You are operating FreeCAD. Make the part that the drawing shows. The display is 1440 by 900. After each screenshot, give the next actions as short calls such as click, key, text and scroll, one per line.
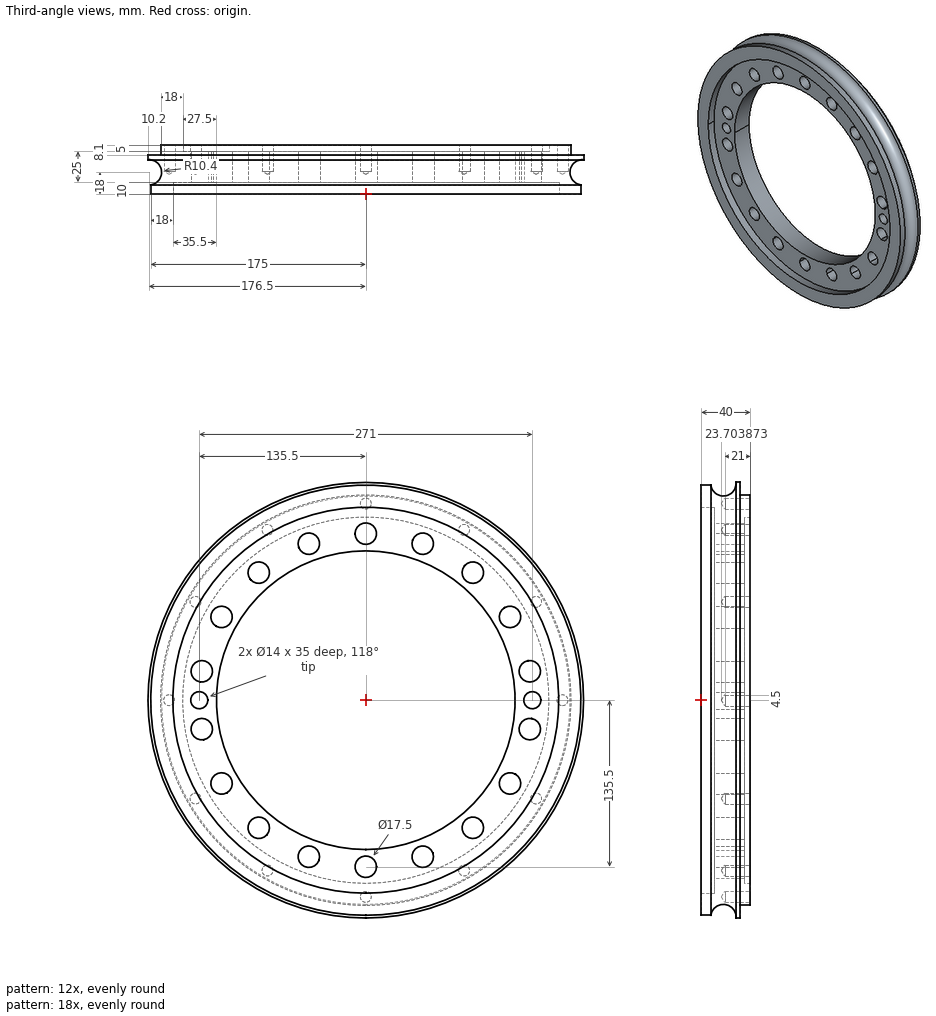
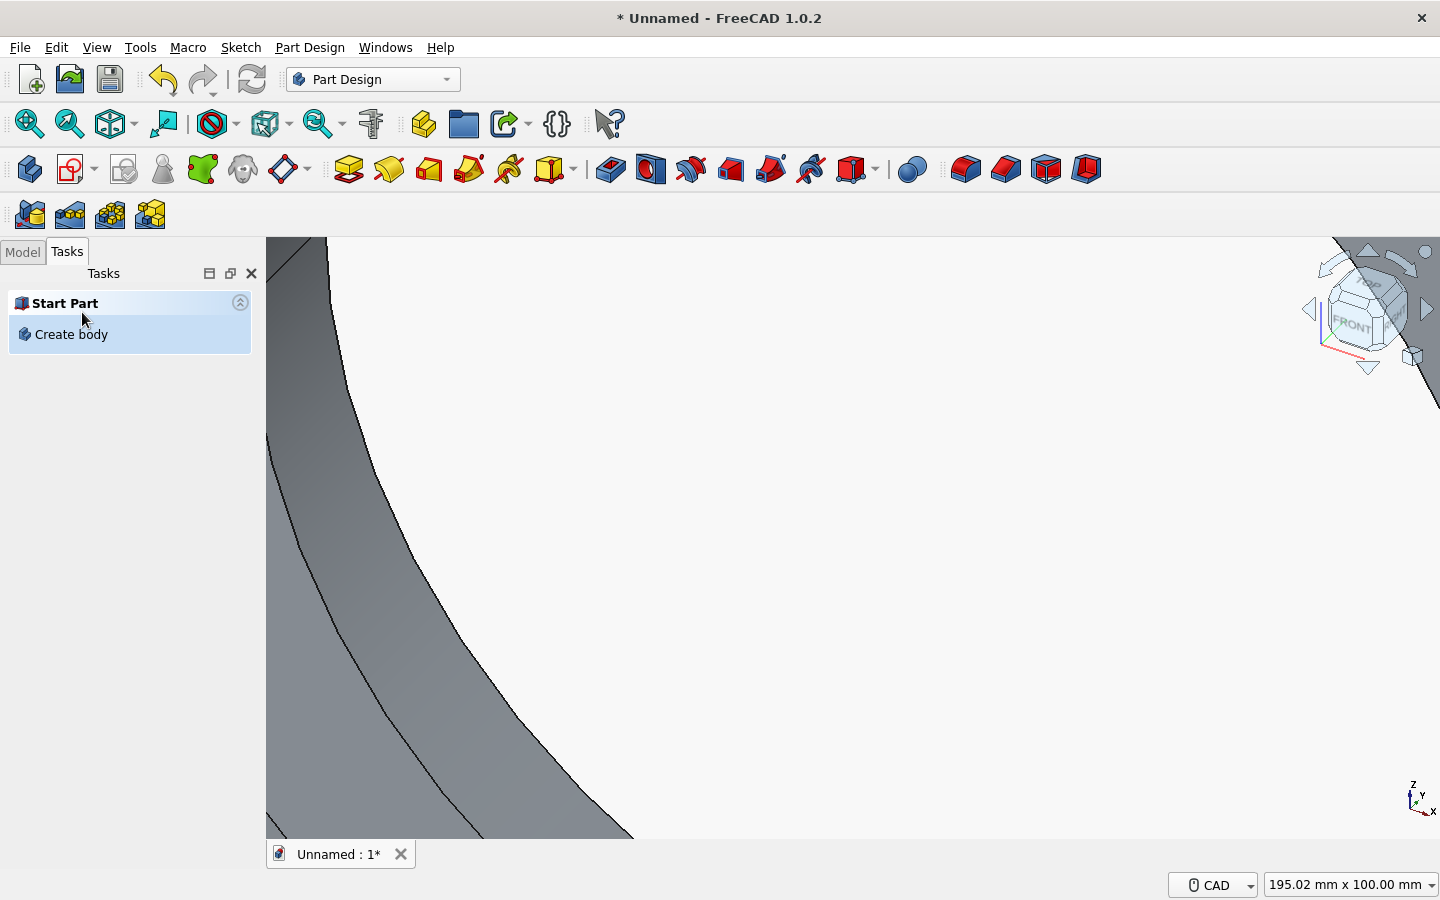
click(30, 124)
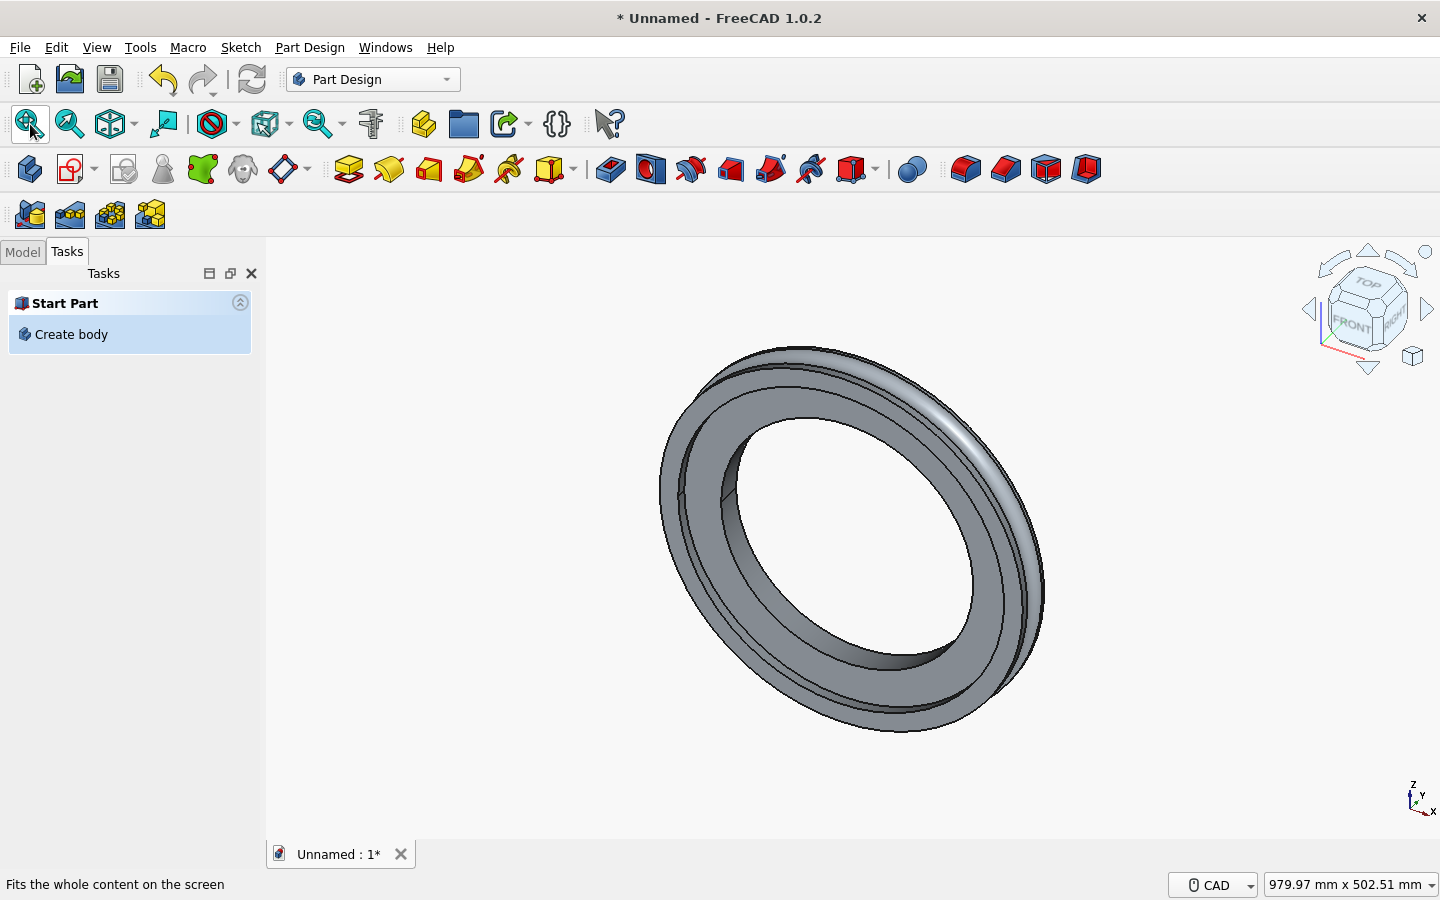
click(23, 251)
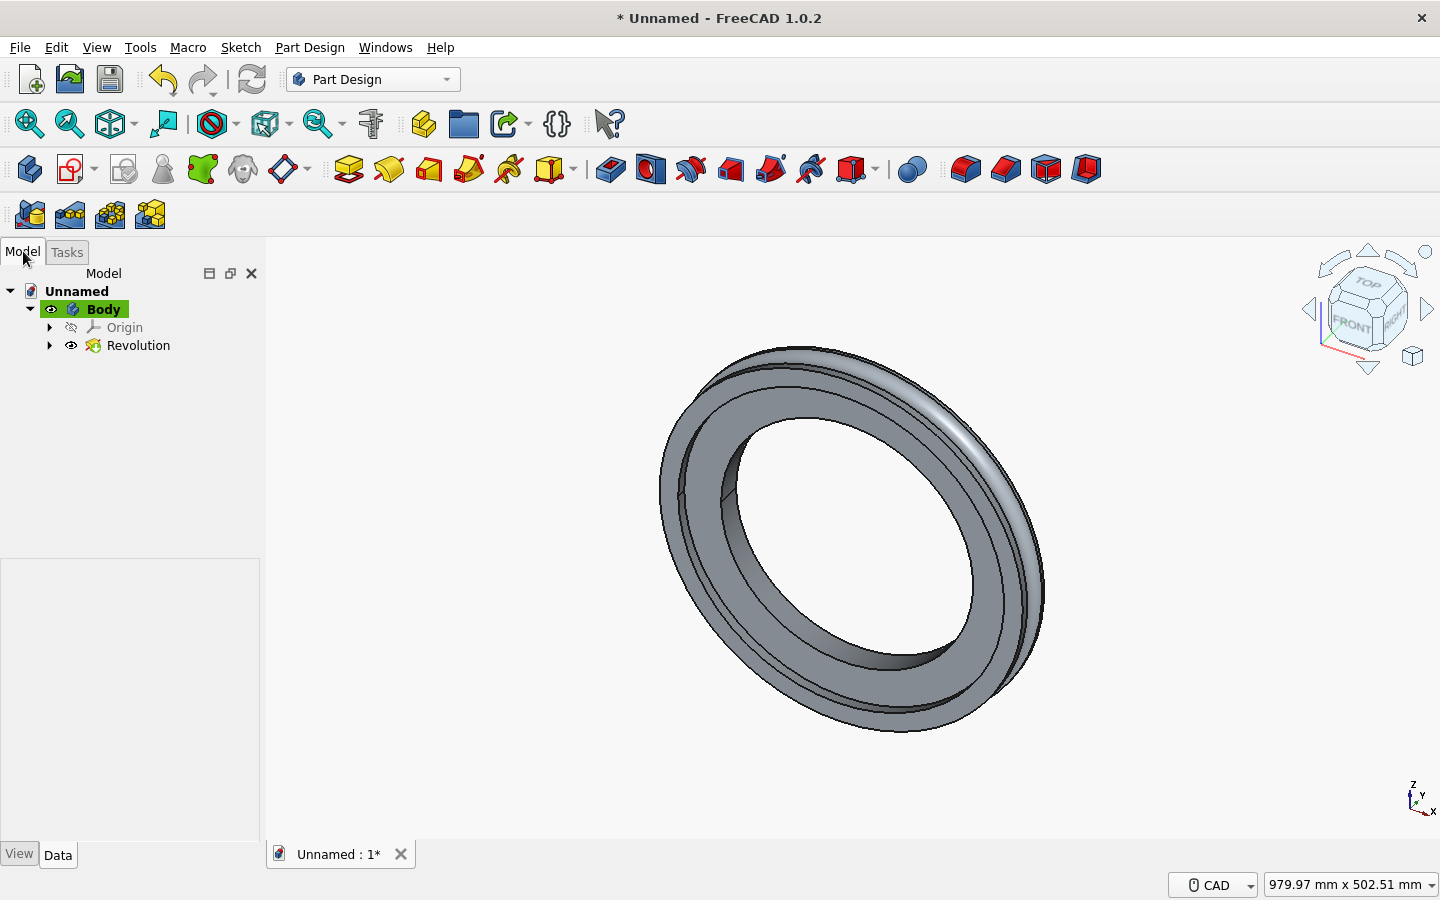
click(50, 327)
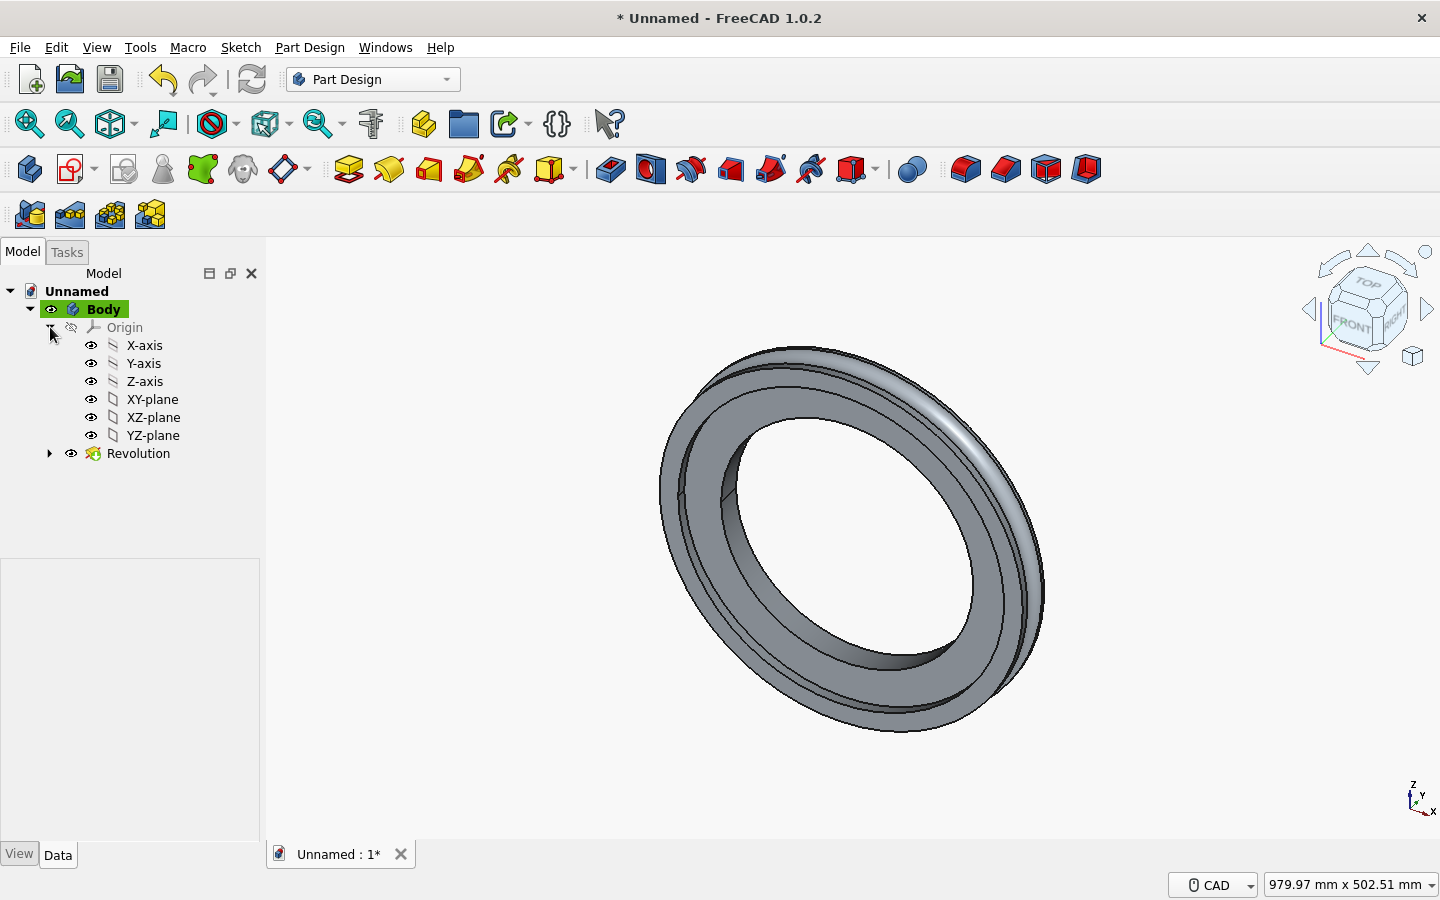
click(136, 435)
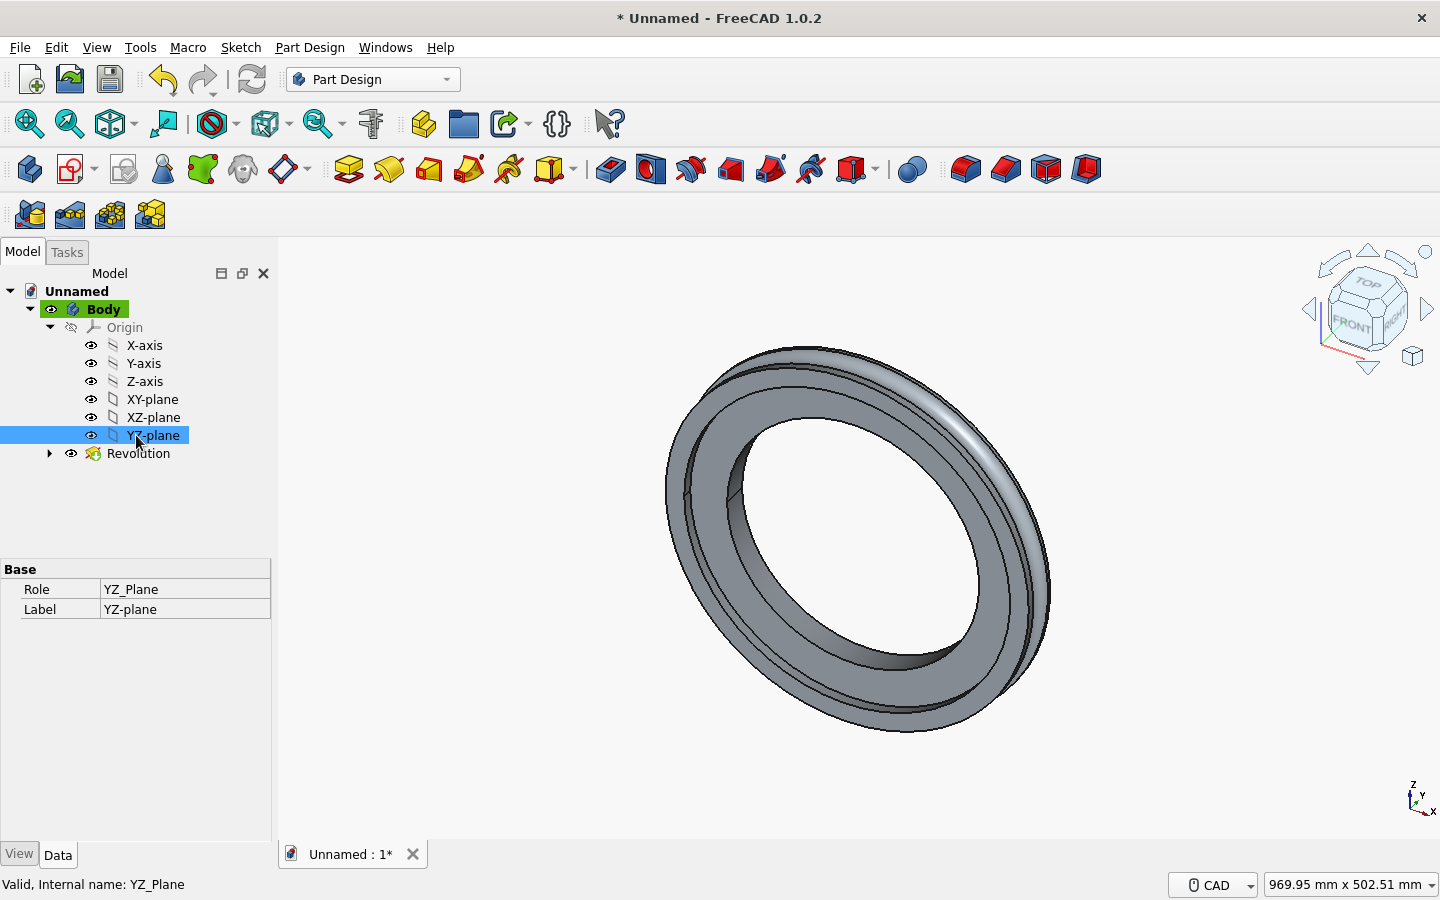
click(284, 170)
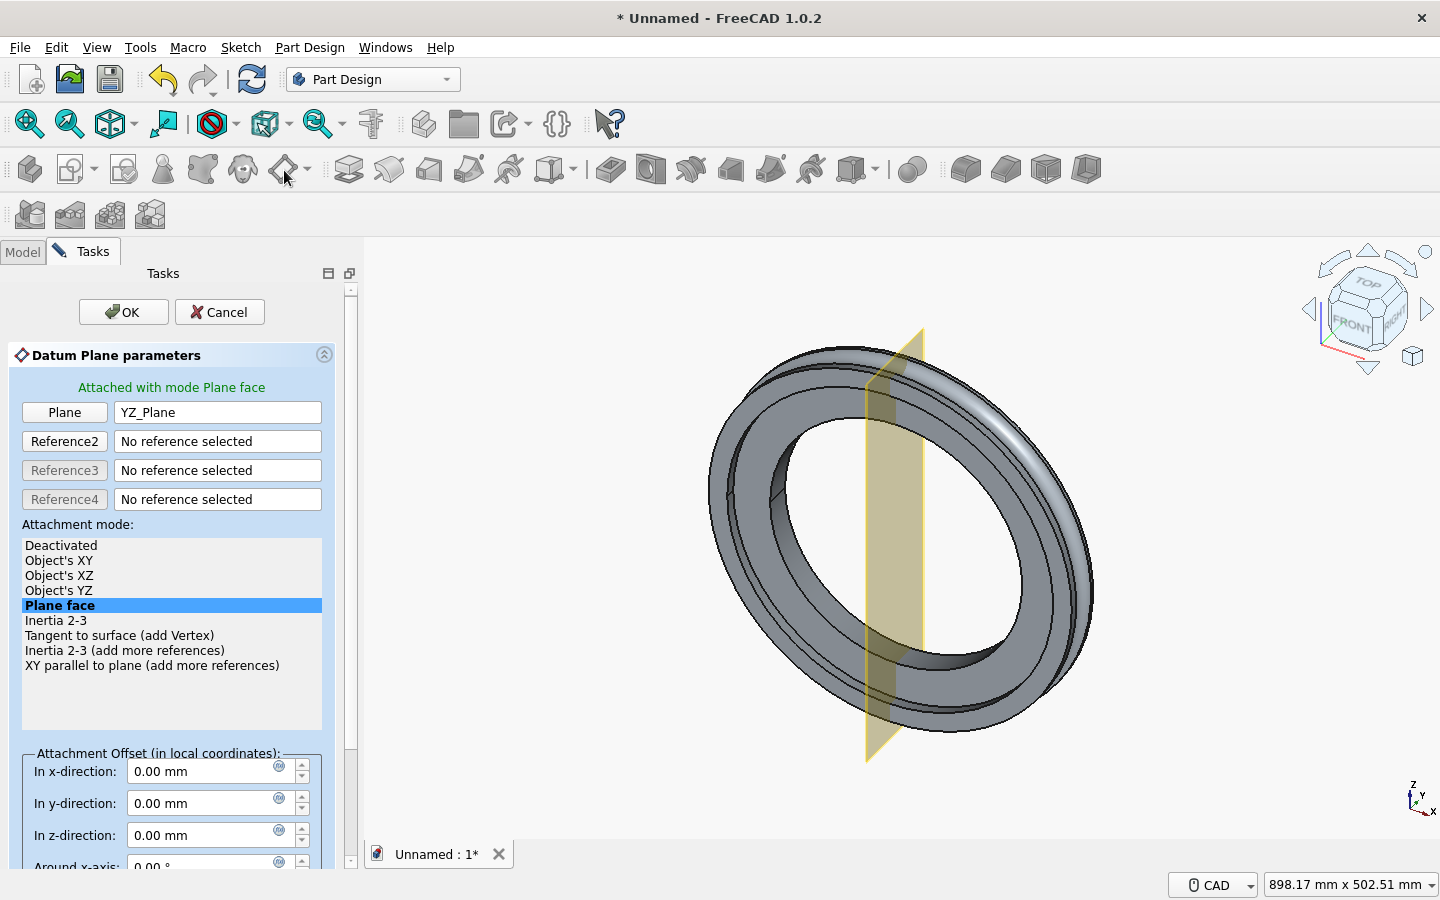
triple_click(210, 835)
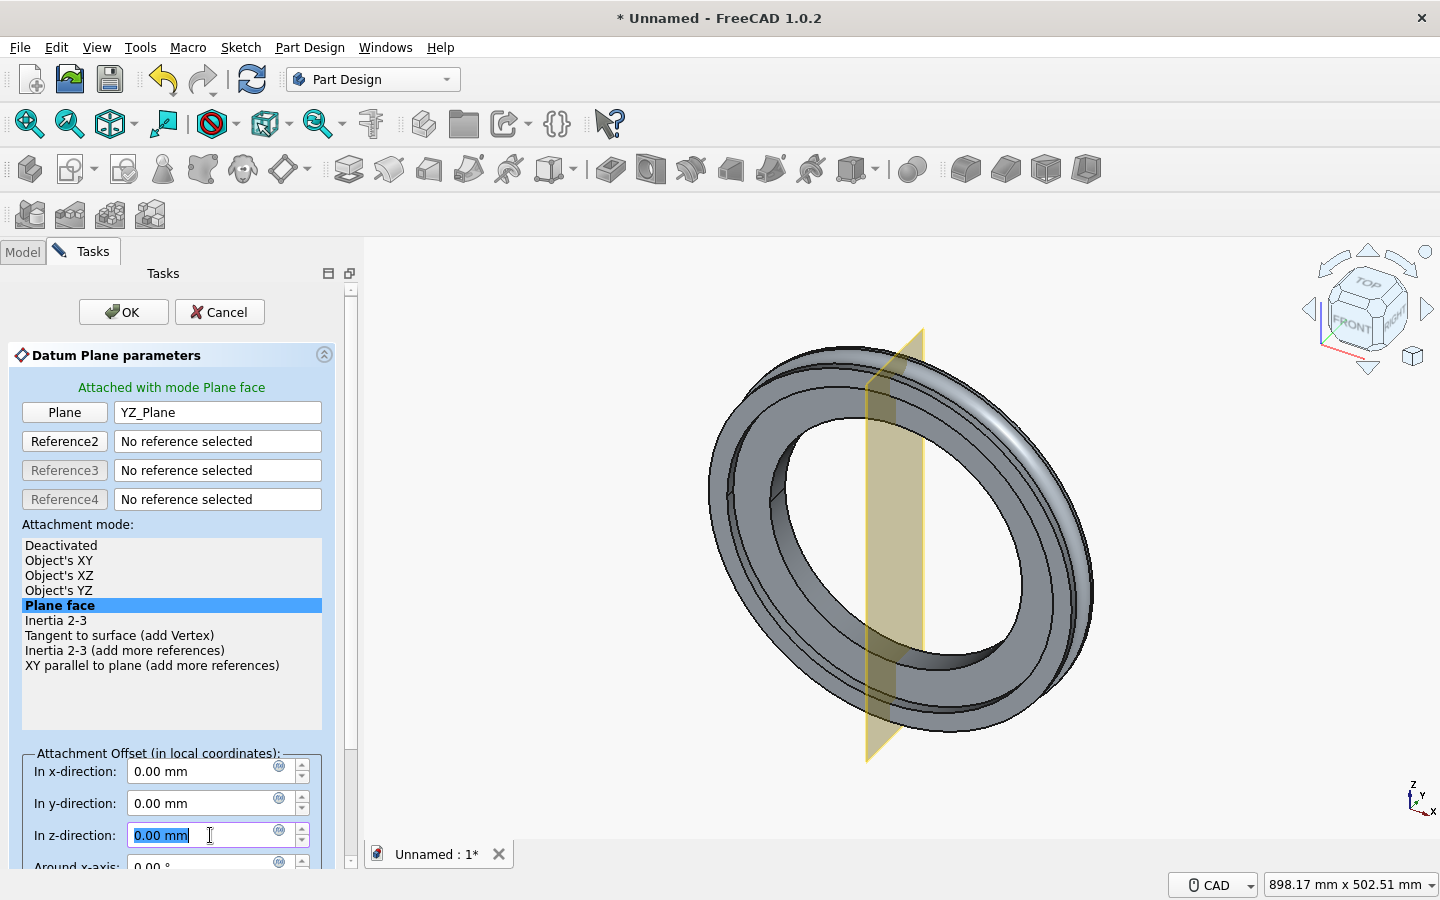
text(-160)
key(Tab)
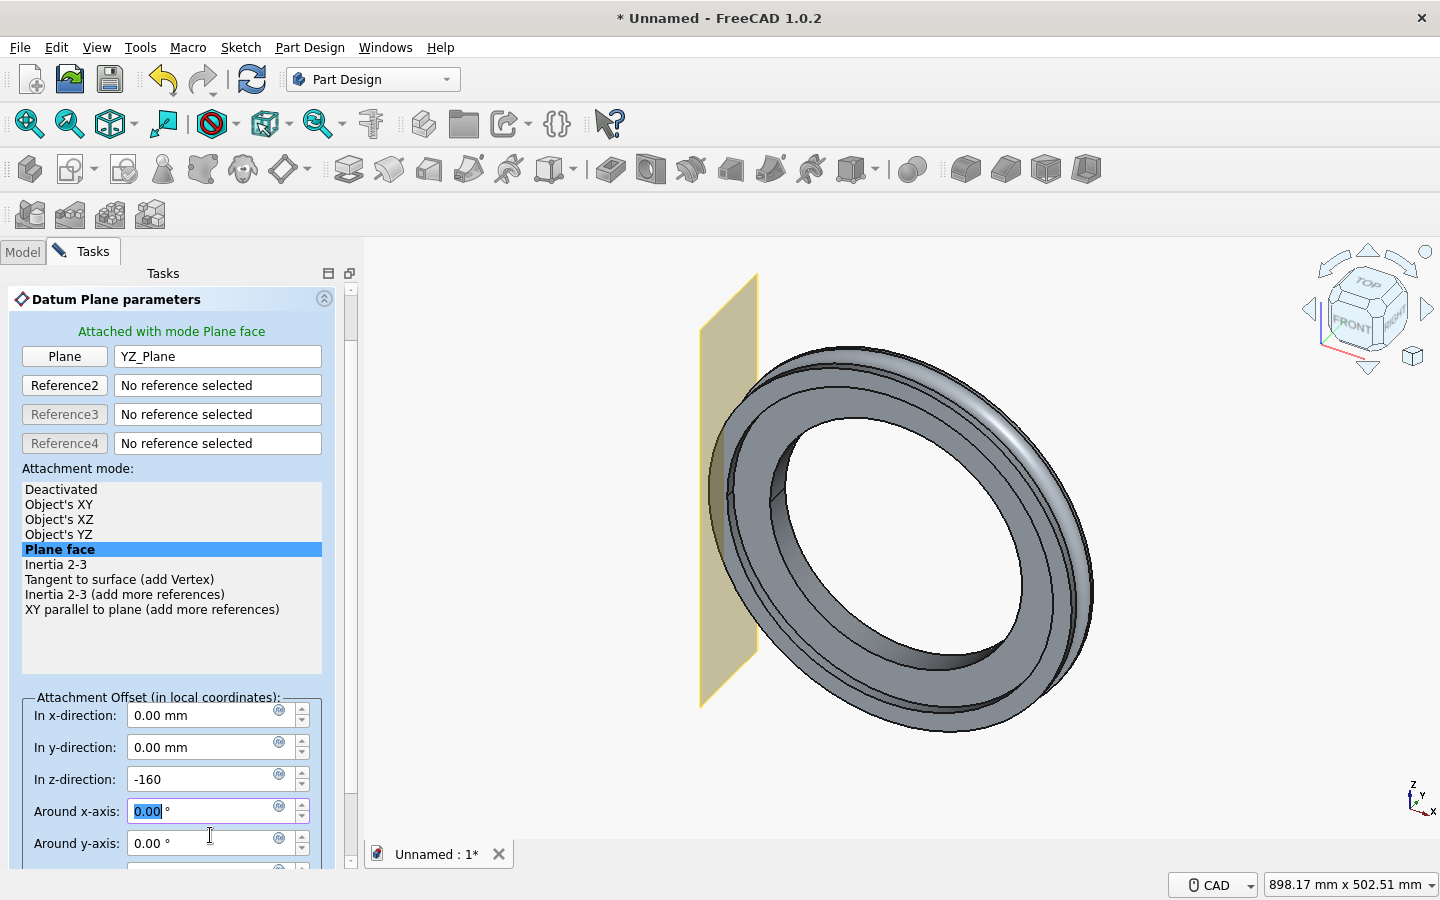
scroll(351, 576, up, 2)